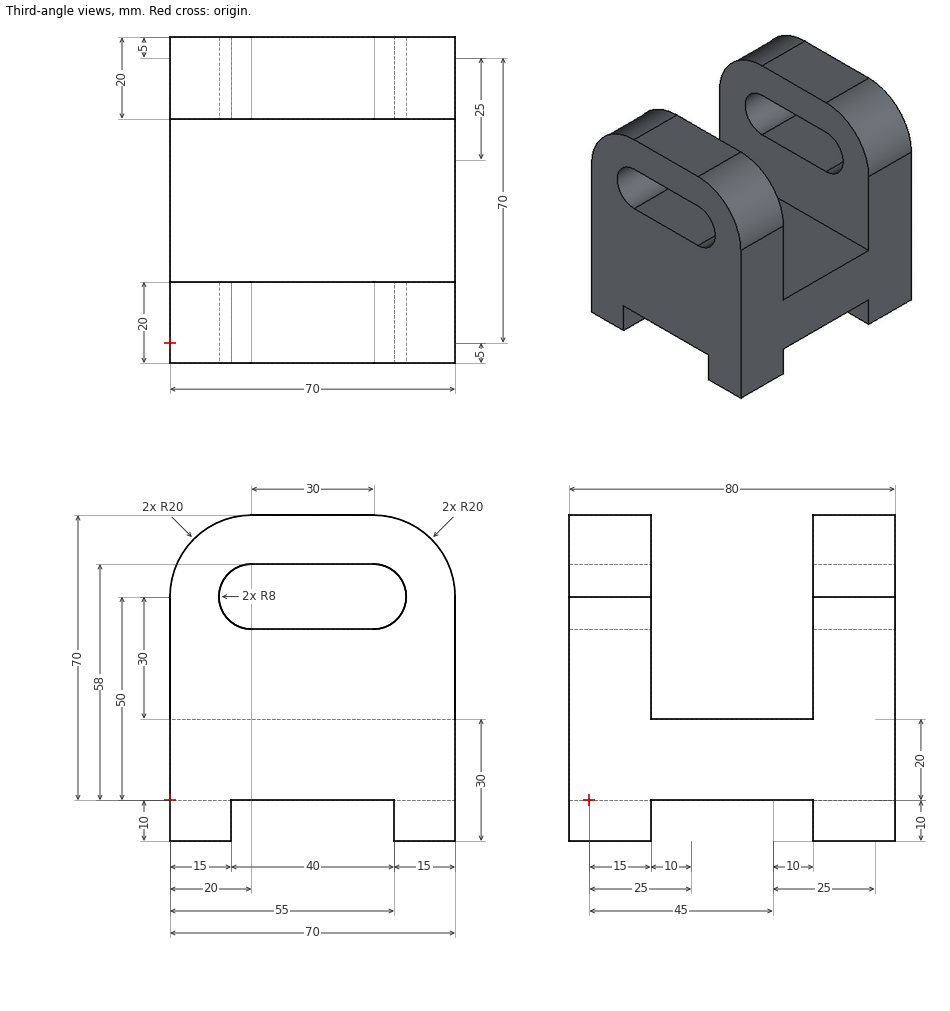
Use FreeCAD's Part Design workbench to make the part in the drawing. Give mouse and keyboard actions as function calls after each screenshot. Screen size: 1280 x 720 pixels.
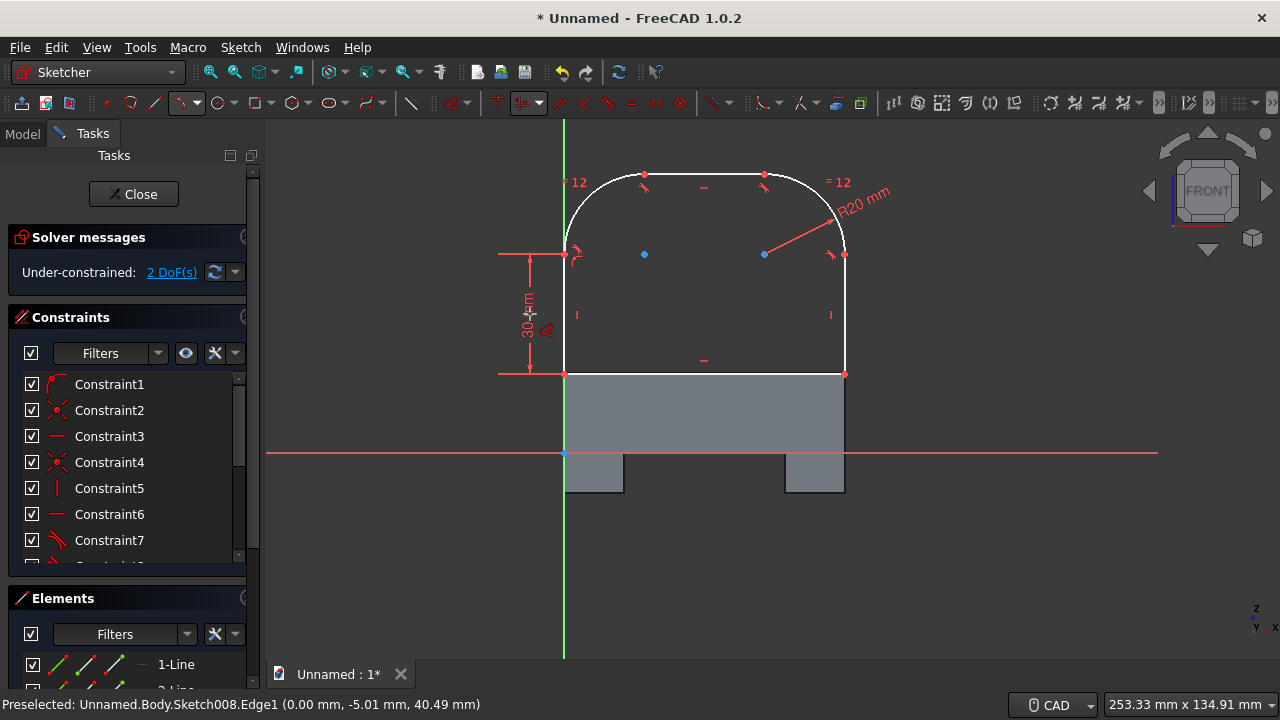
click(649, 374)
click(705, 408)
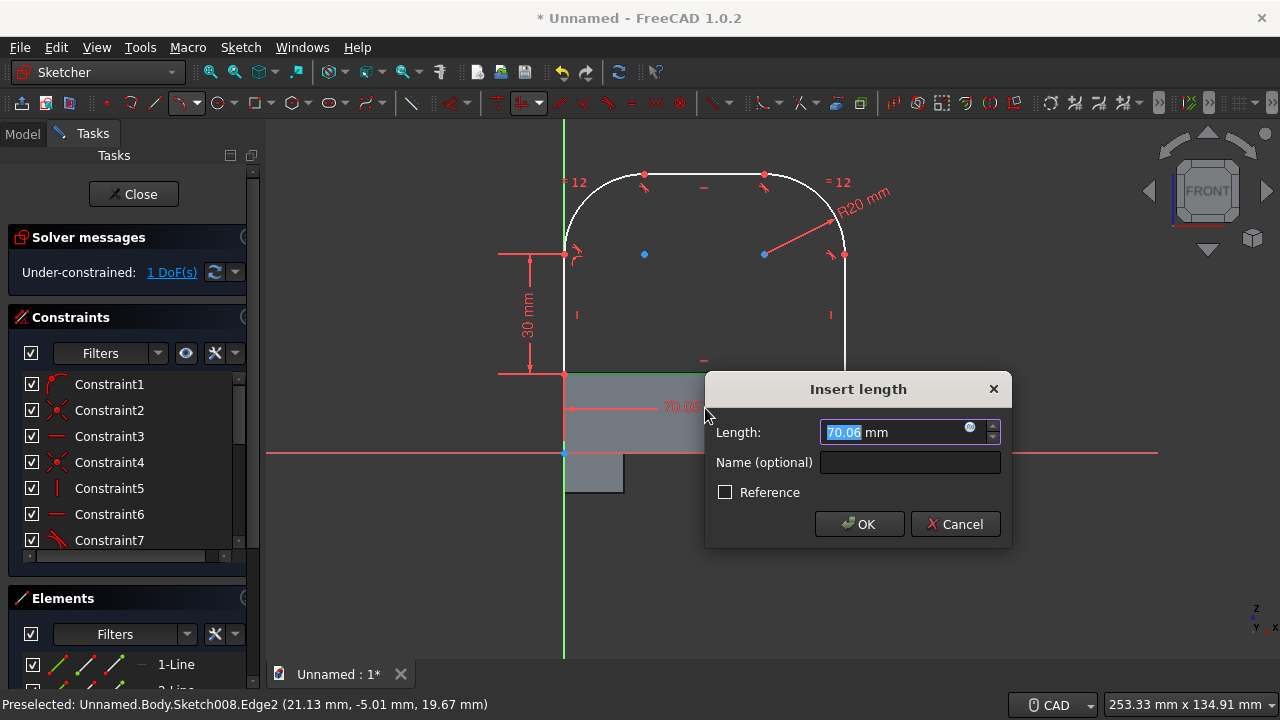
text(70)
key(Return)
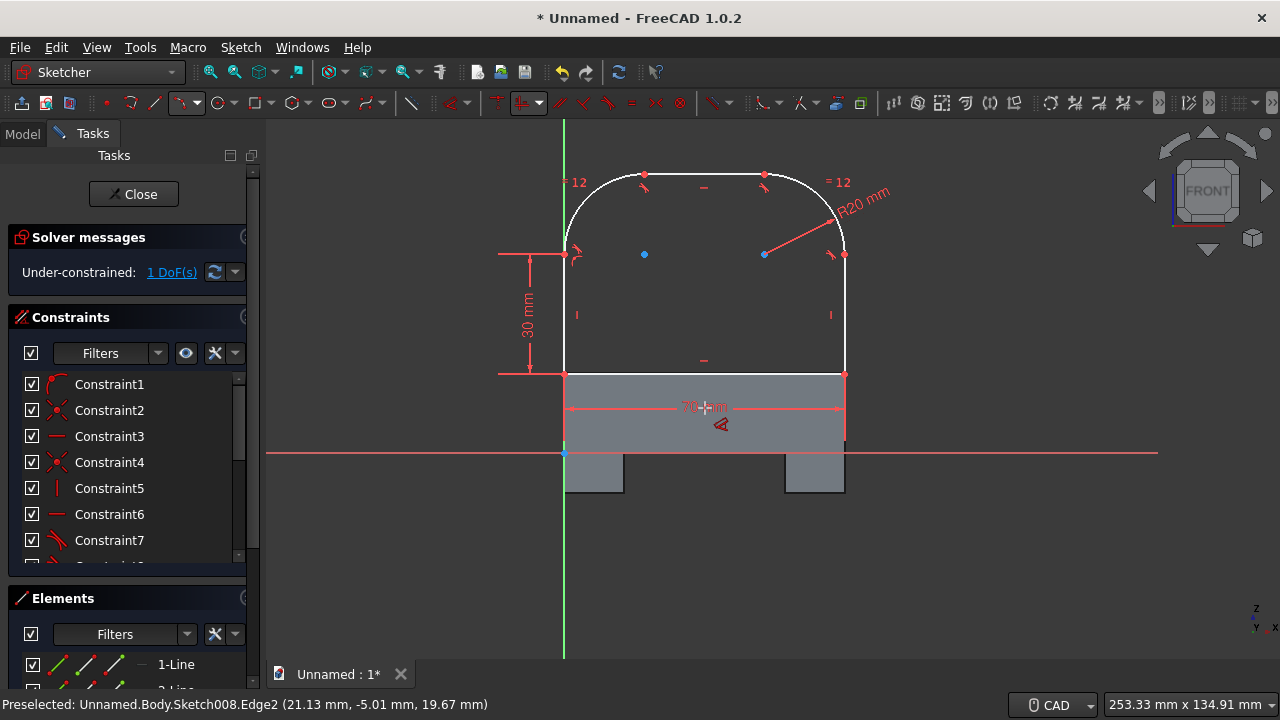
click(564, 254)
click(530, 354)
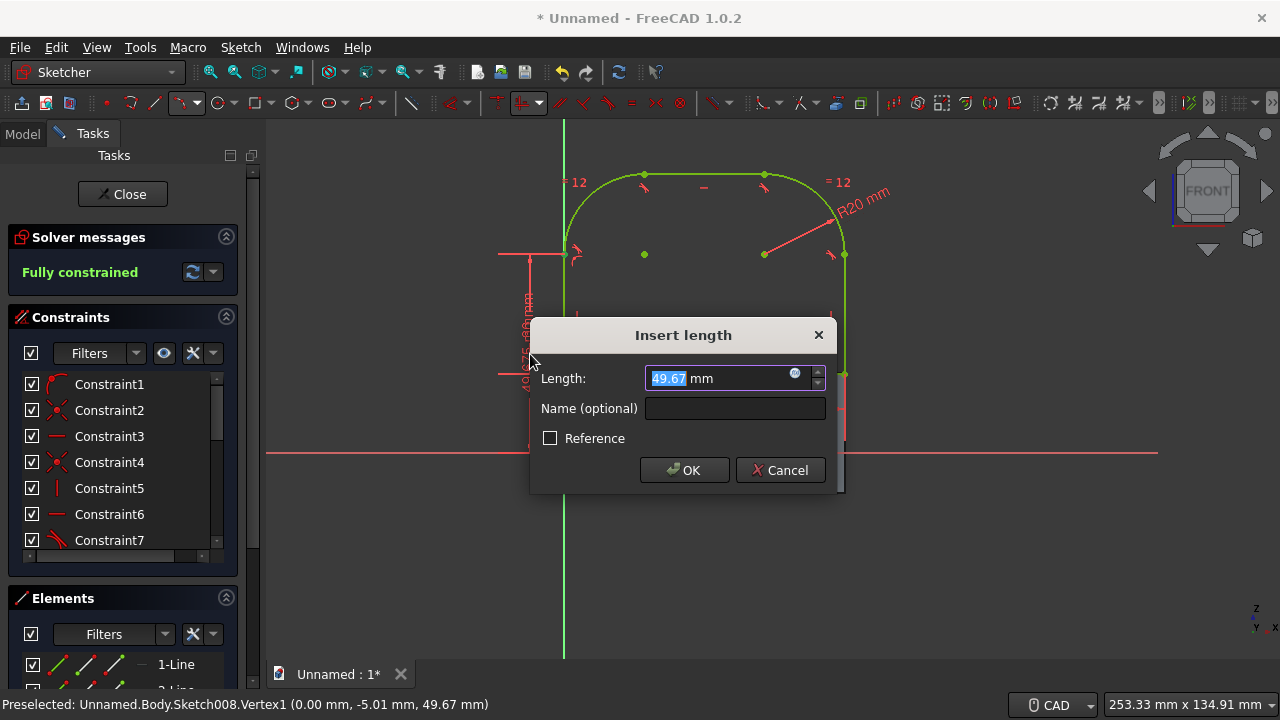
text(50)
key(Return)
key(Escape)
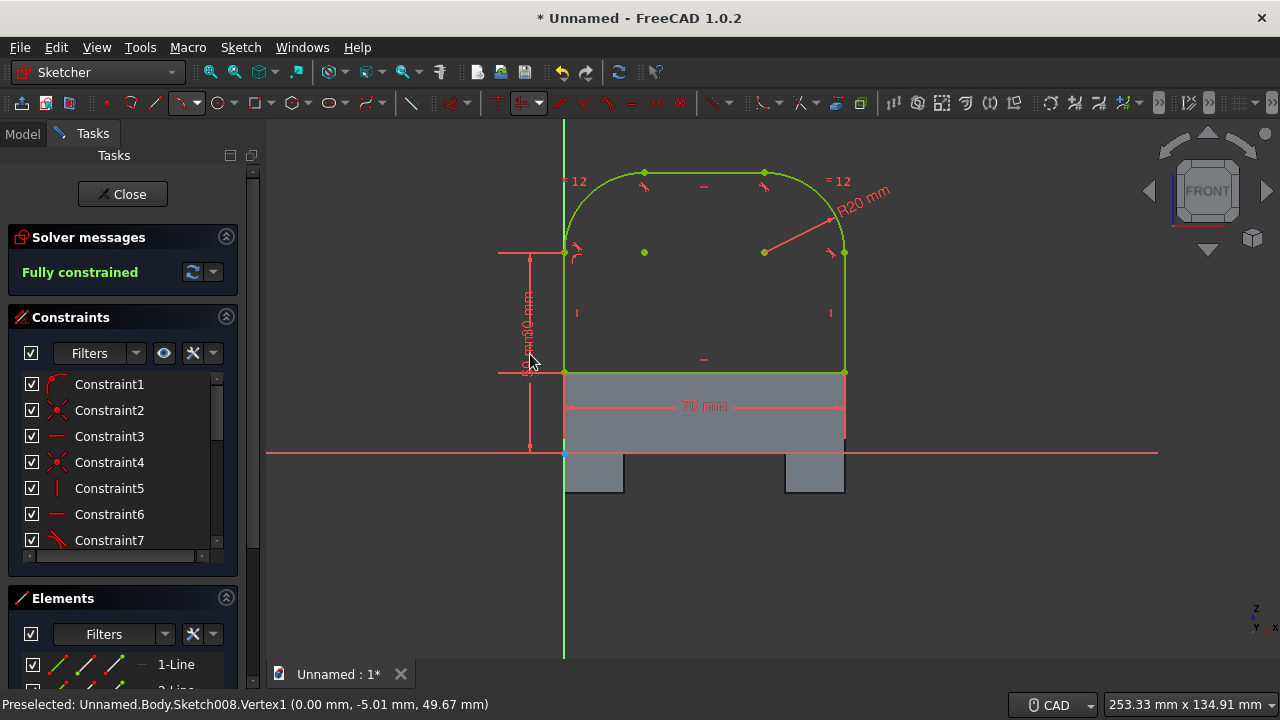
click(123, 194)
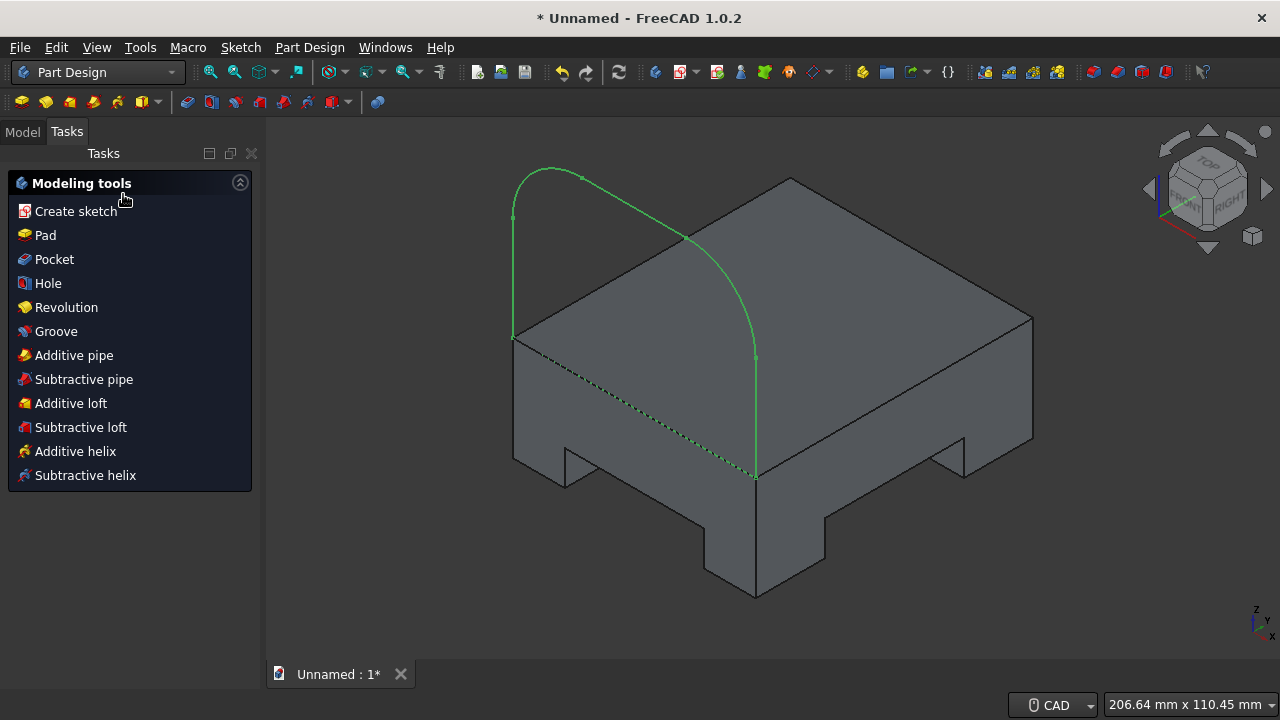
click(22, 102)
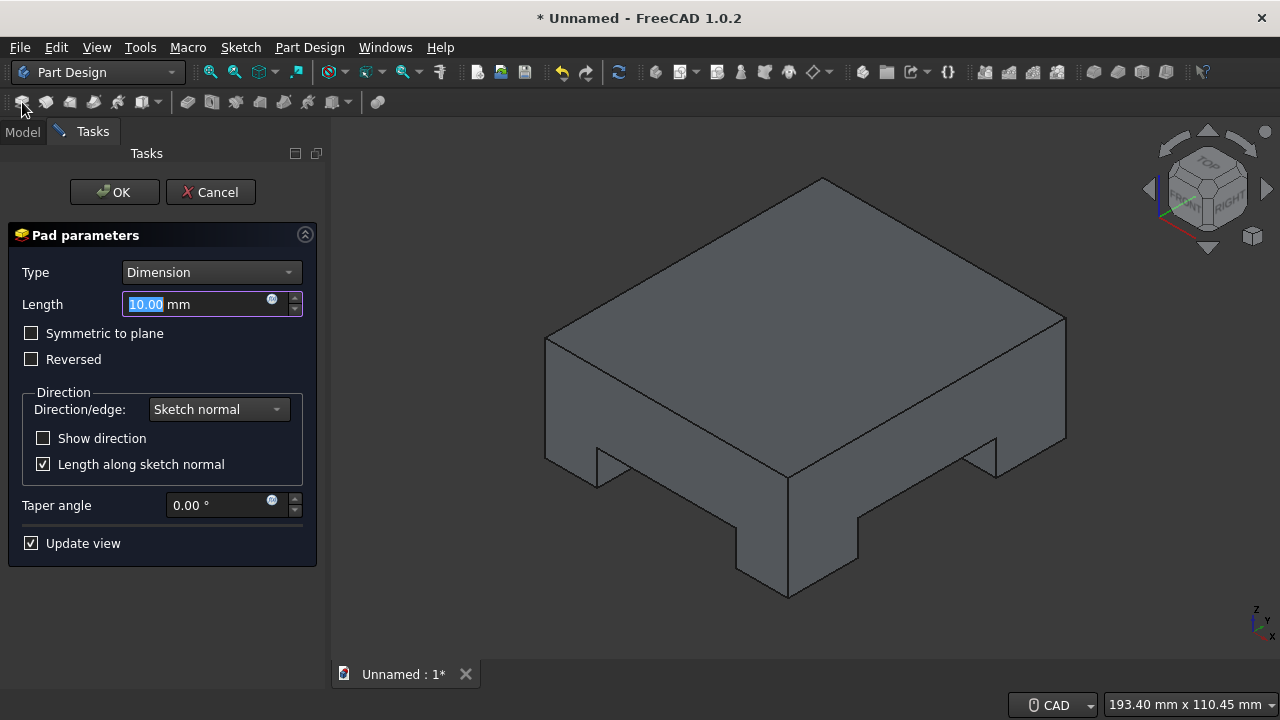
text(20)
key(Tab)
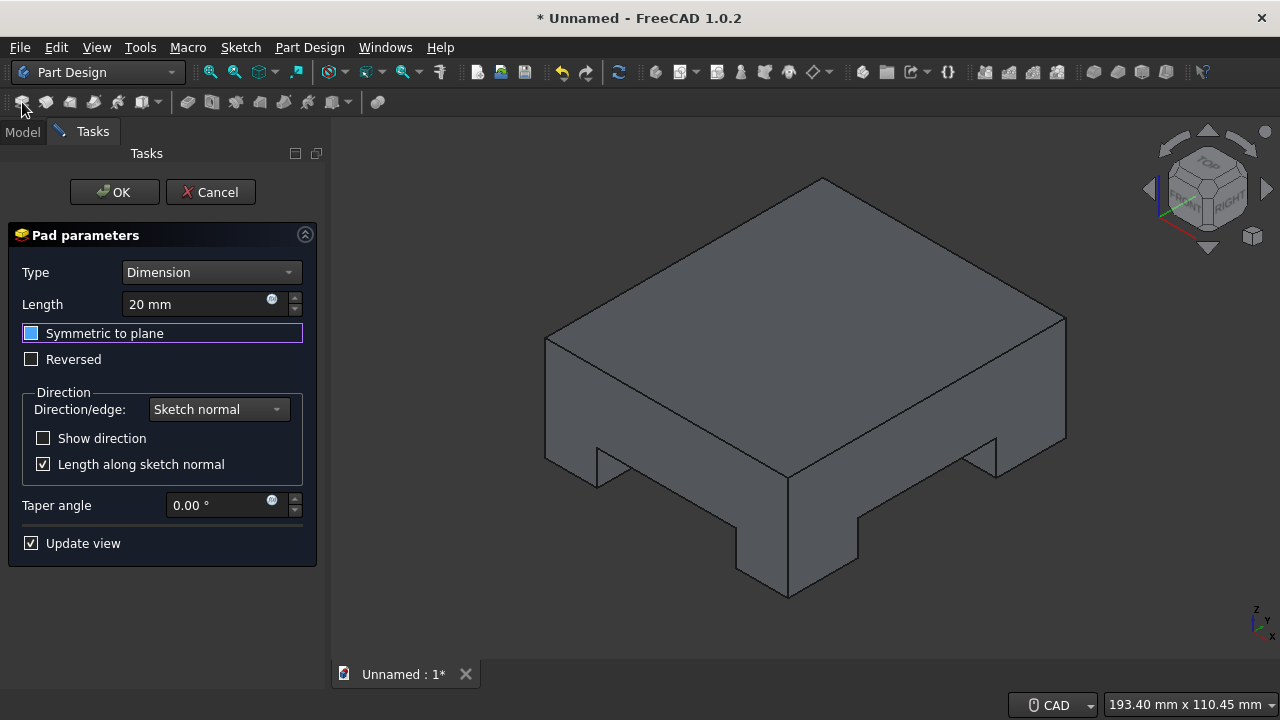
click(30, 359)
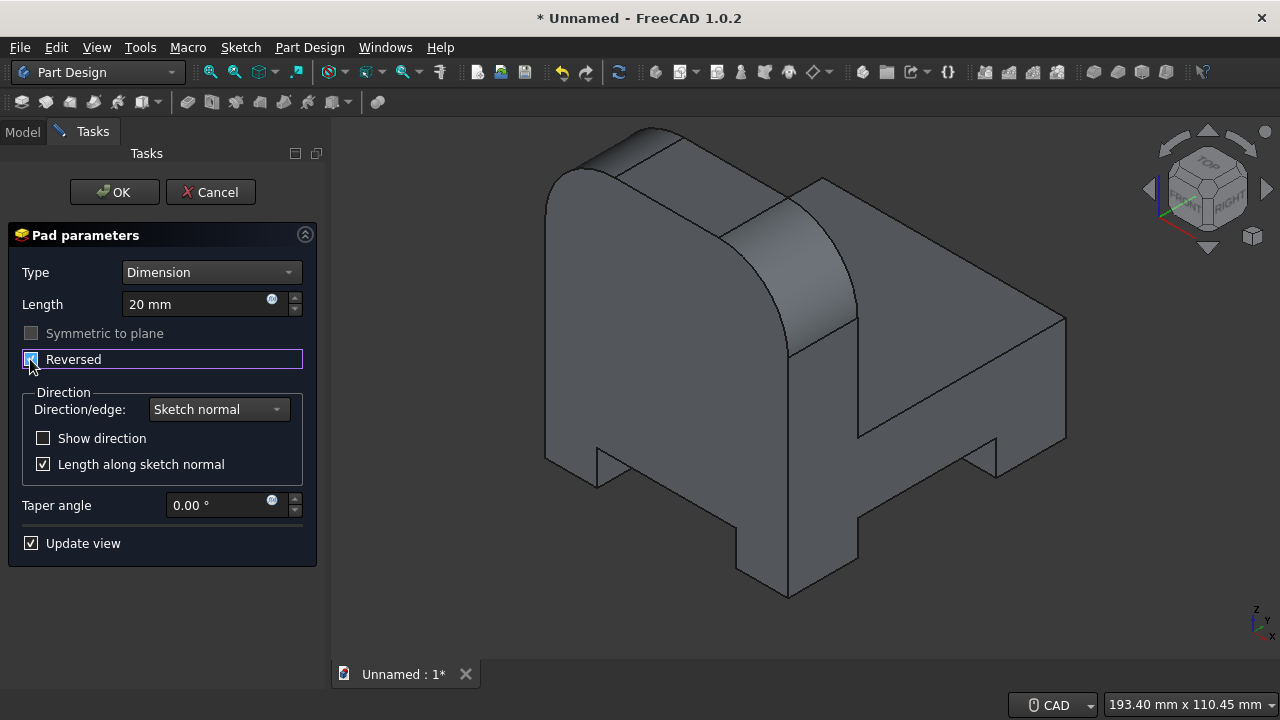
click(115, 192)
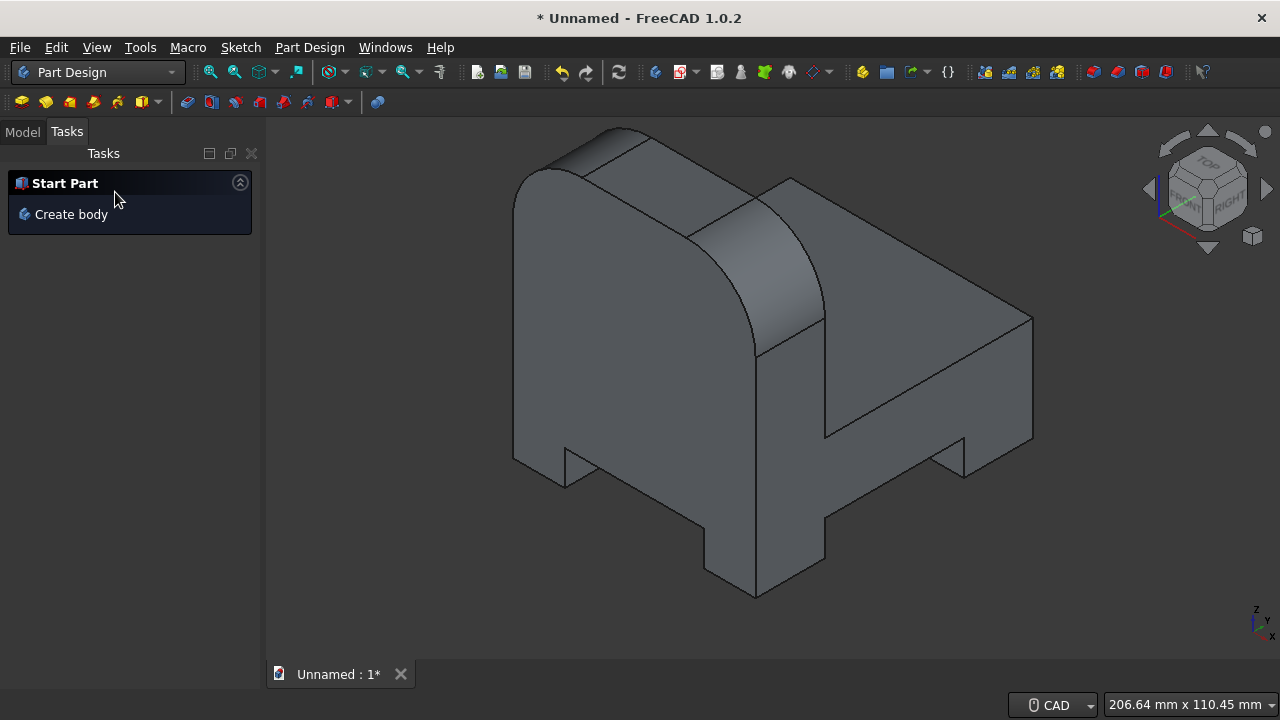
key(v)
key(f)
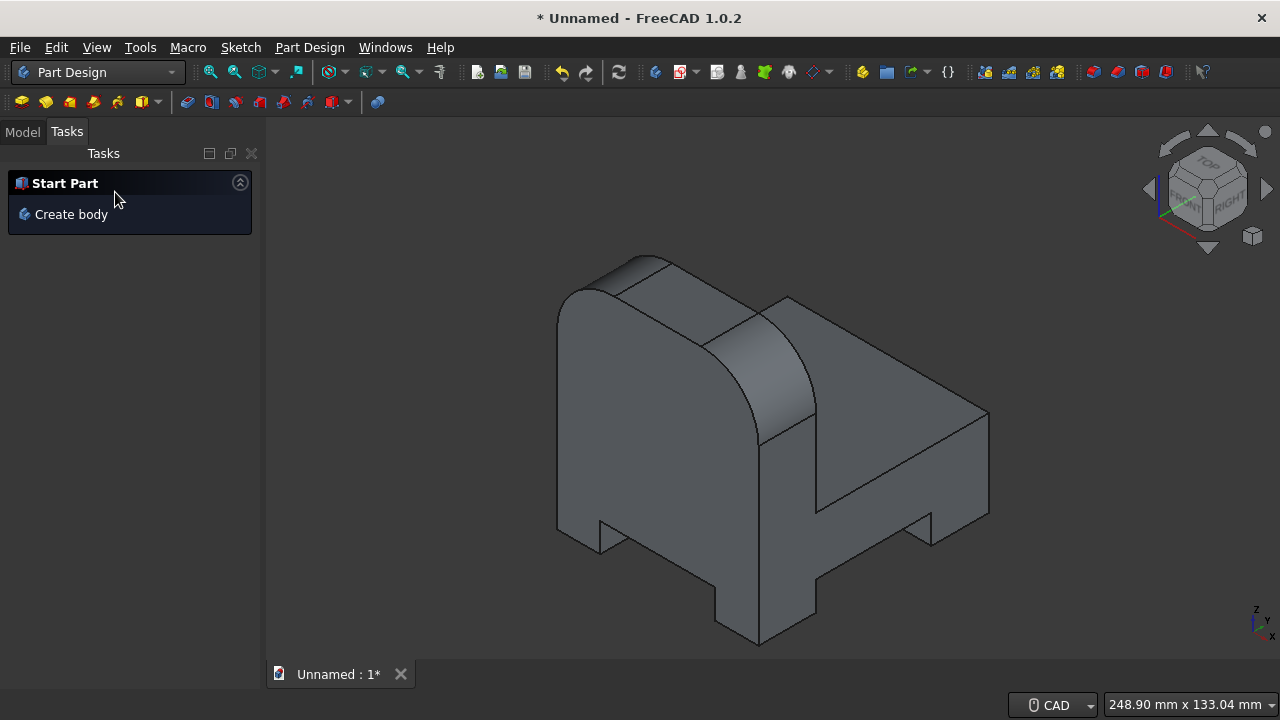
click(23, 131)